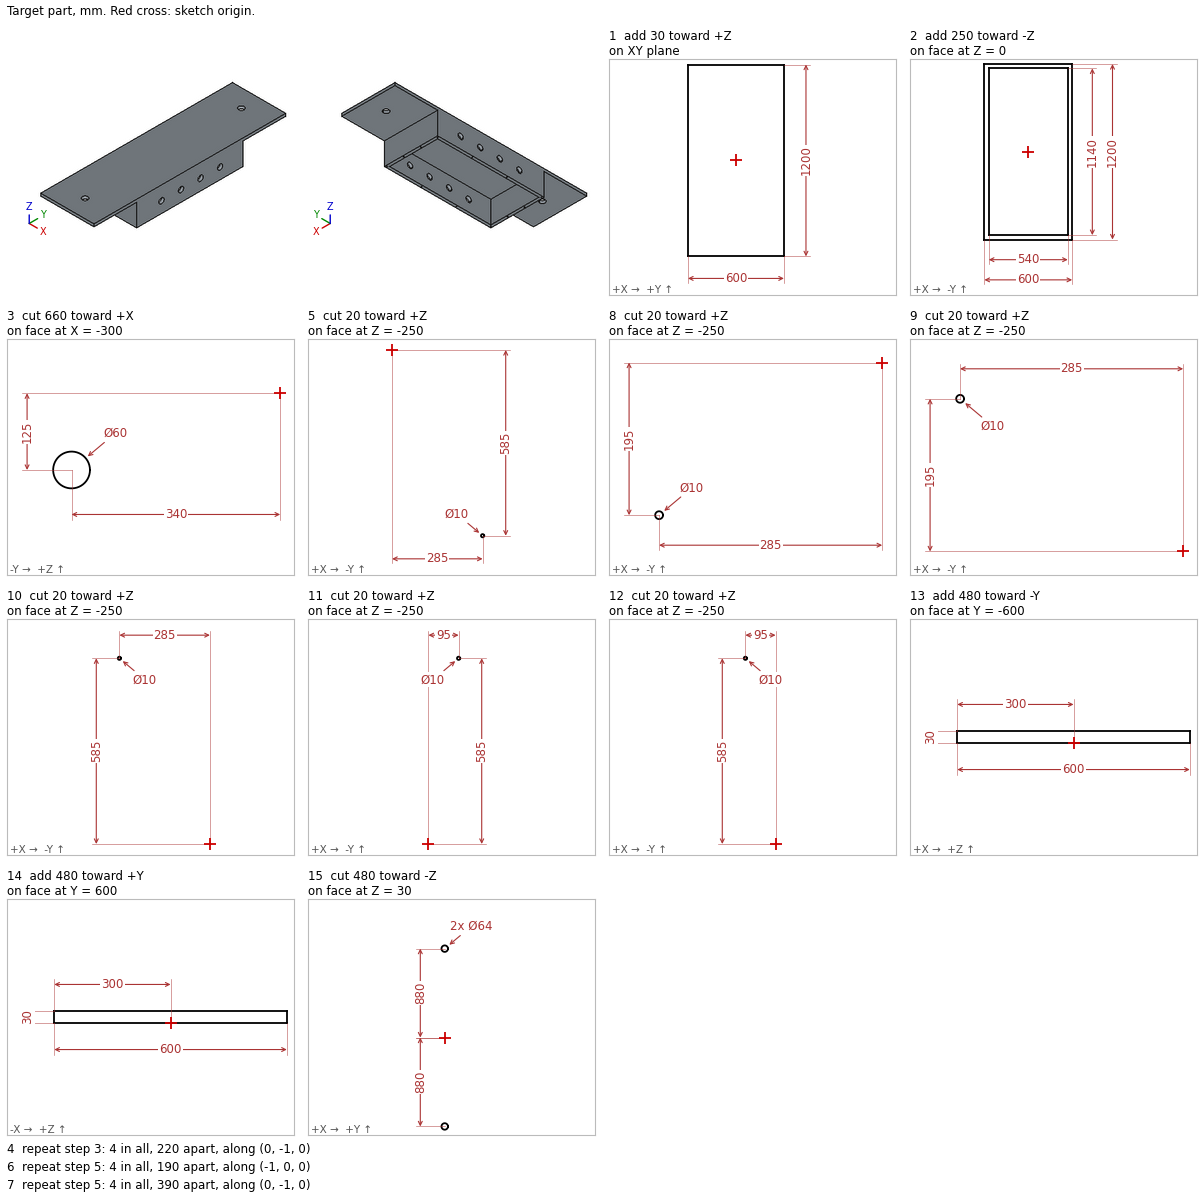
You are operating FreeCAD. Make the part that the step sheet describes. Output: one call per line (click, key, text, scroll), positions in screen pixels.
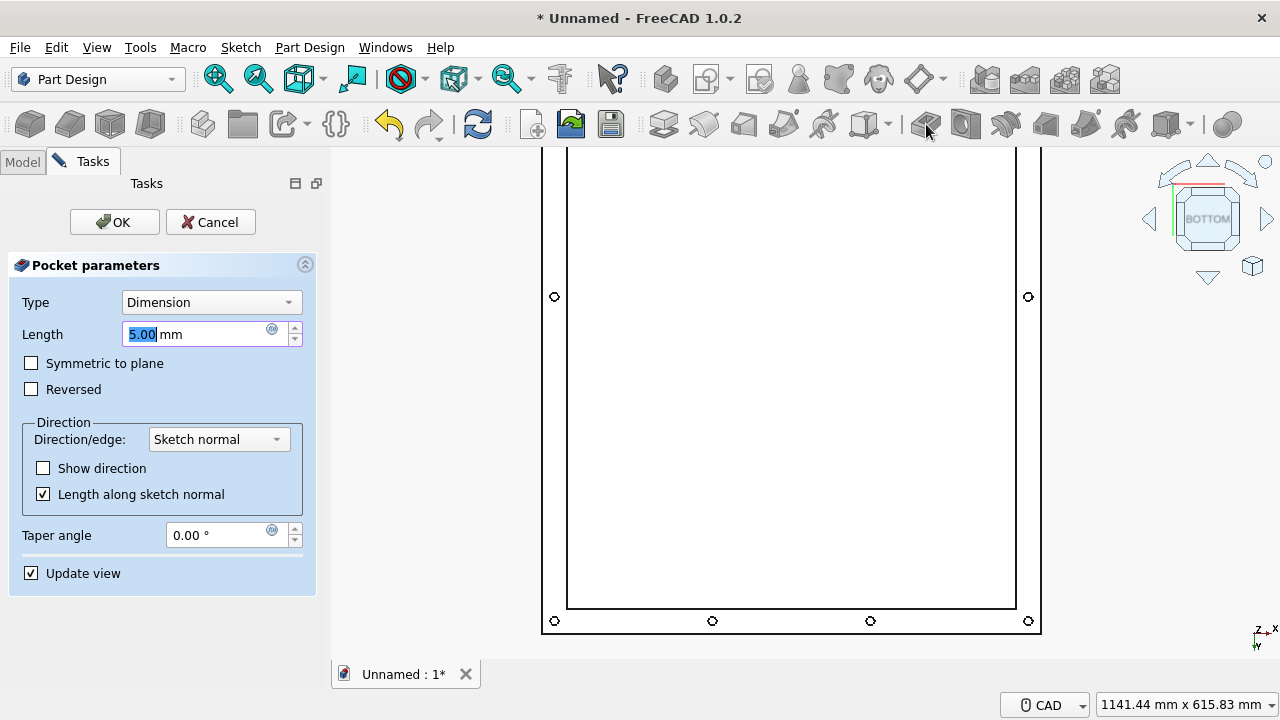
text(20)
key(Tab)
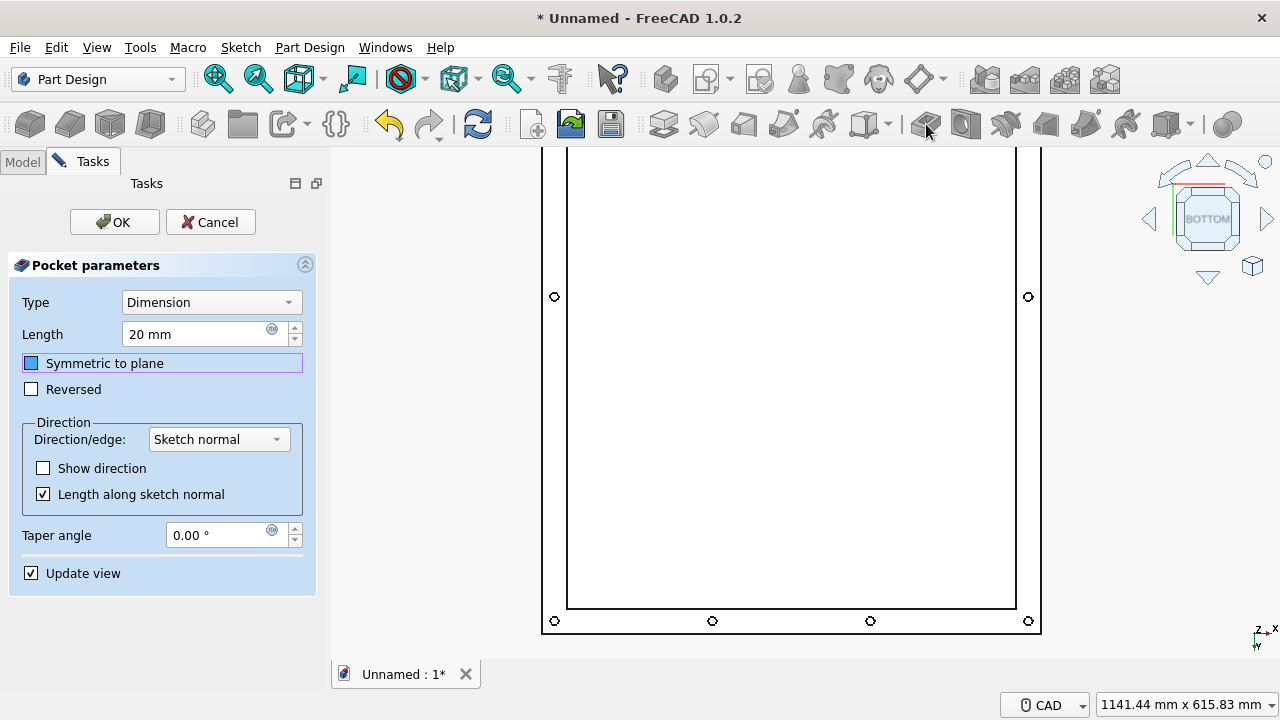
click(115, 222)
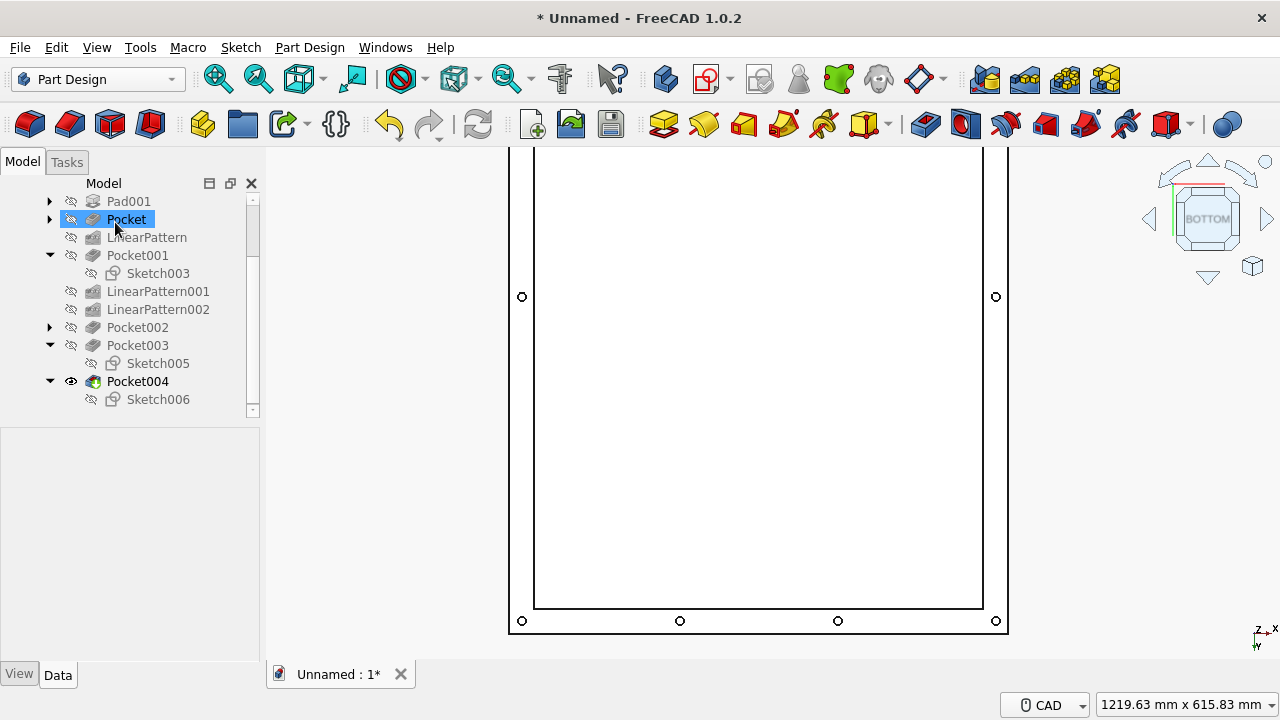
click(220, 80)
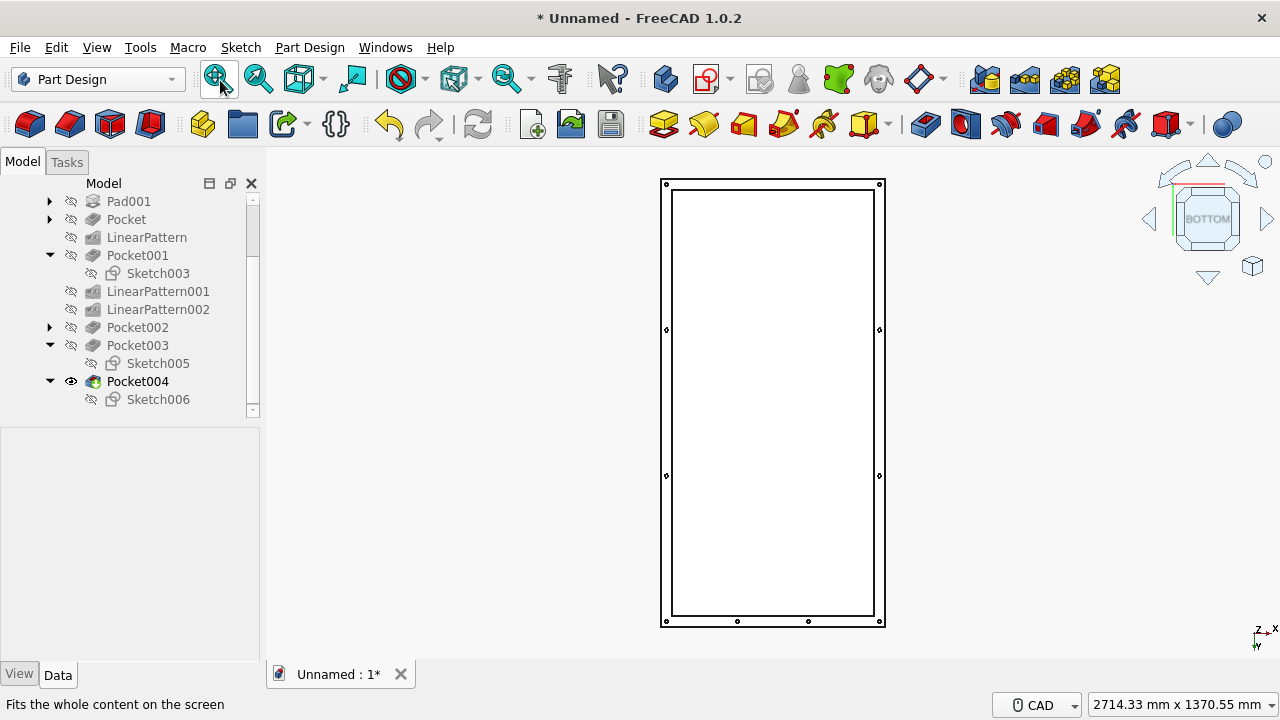
scroll(762, 620, up, 5)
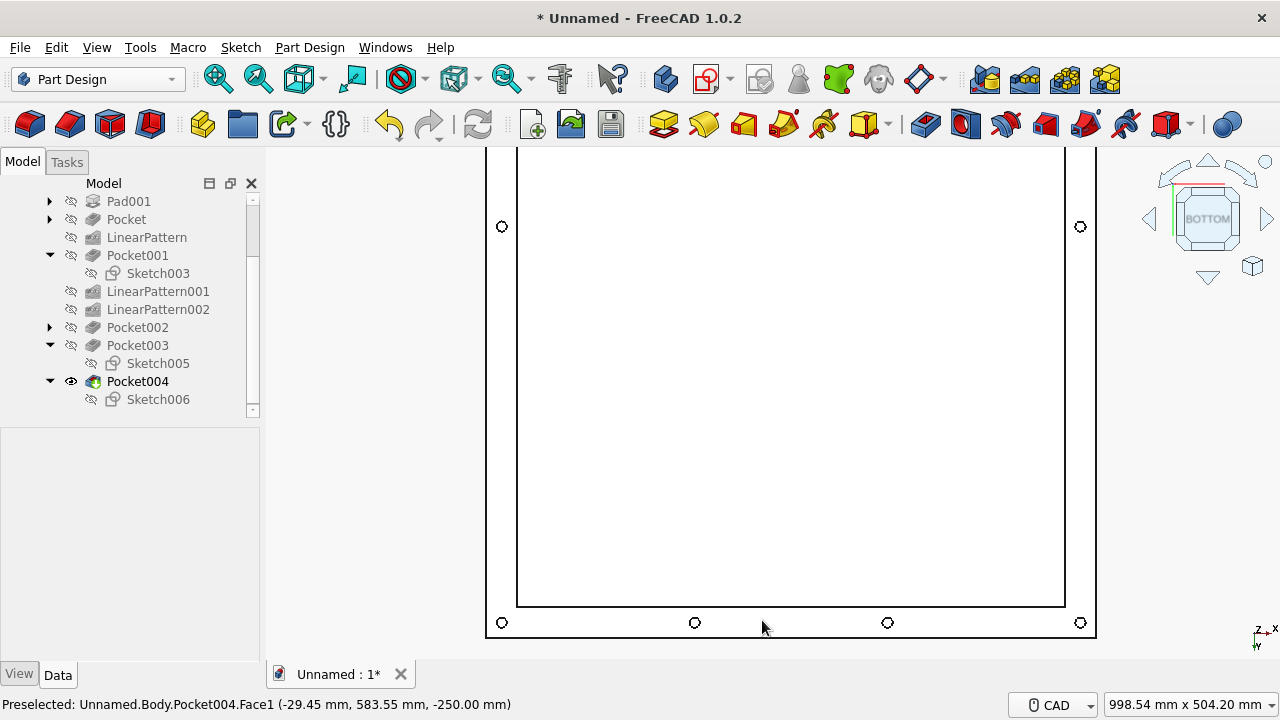
click(760, 621)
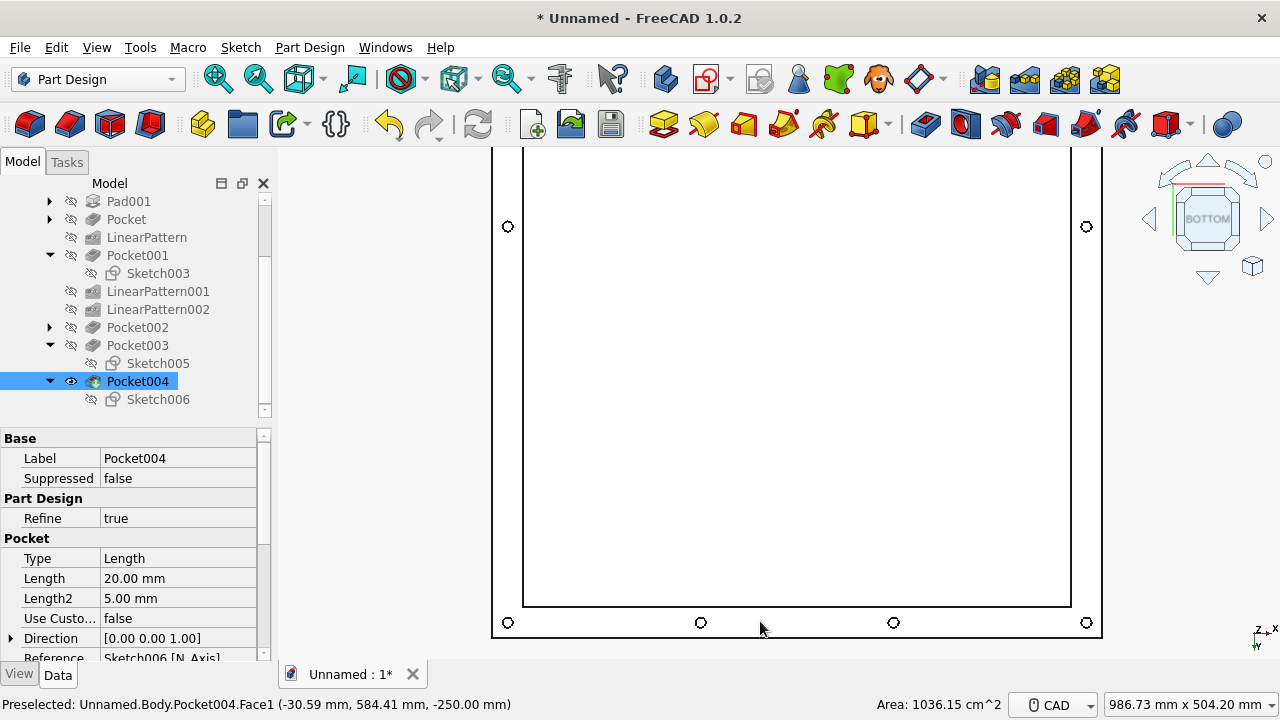
click(706, 80)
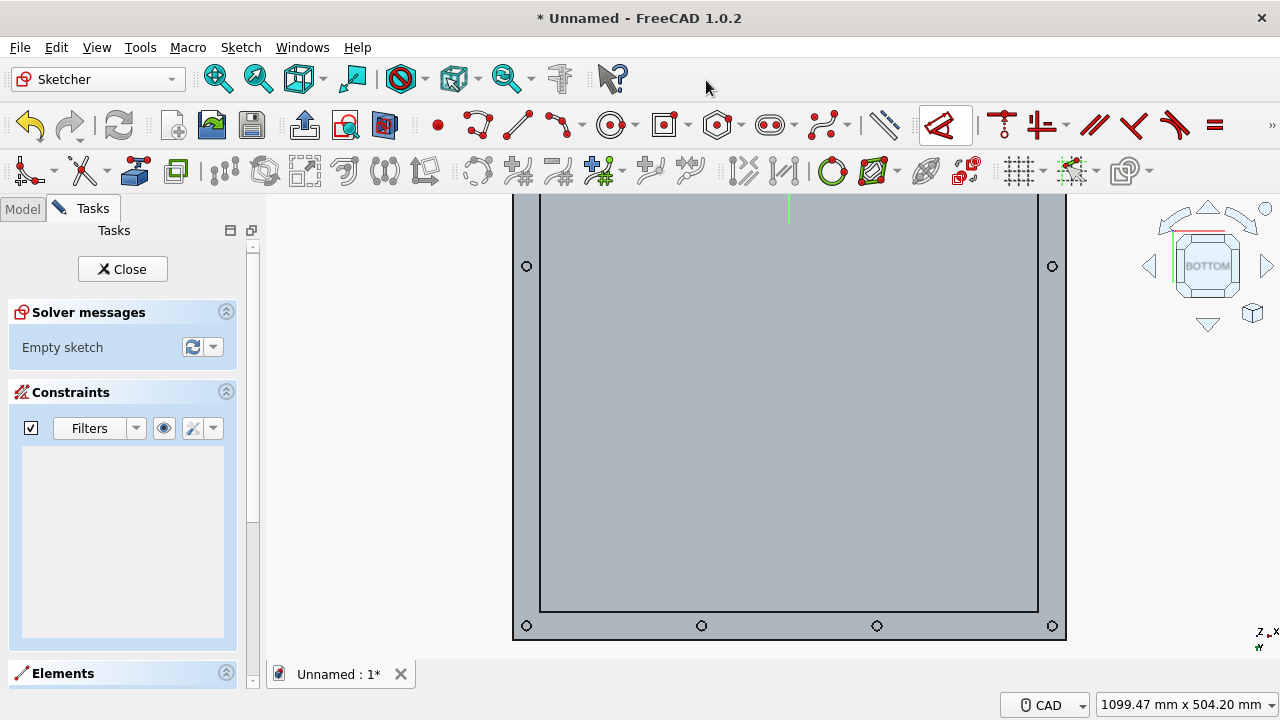
scroll(704, 426, down, 5)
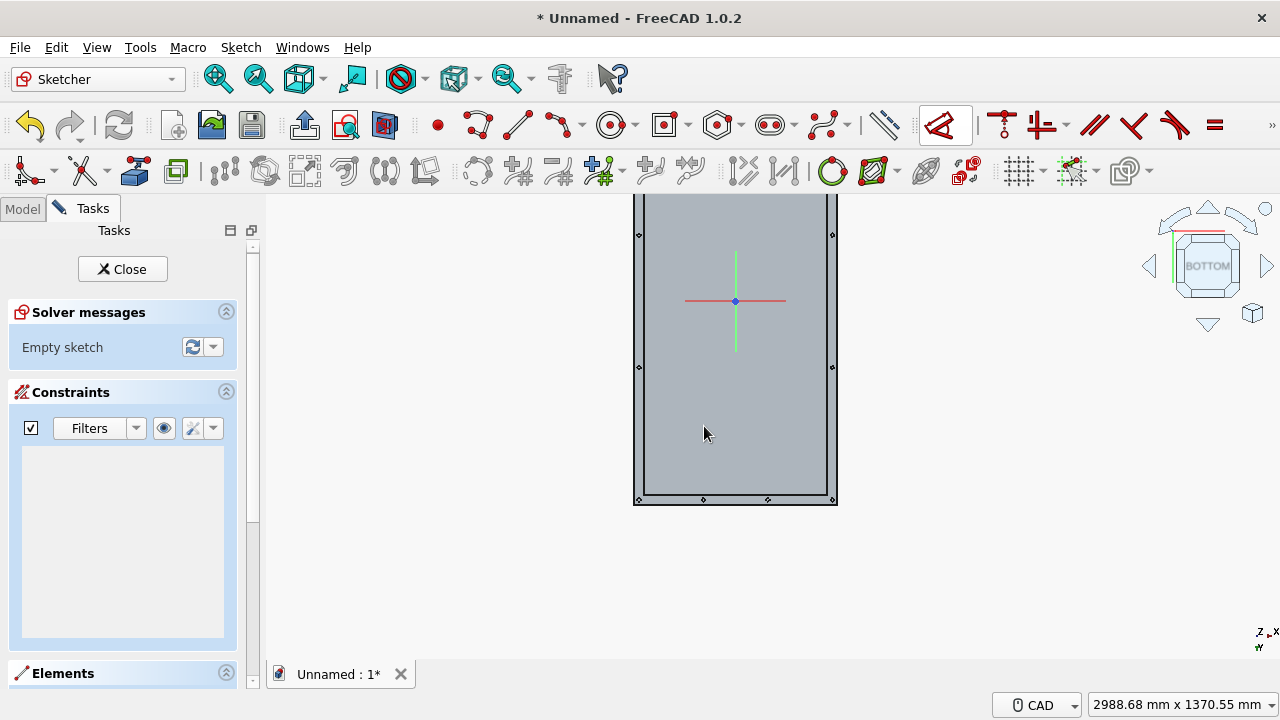
scroll(704, 426, down, 5)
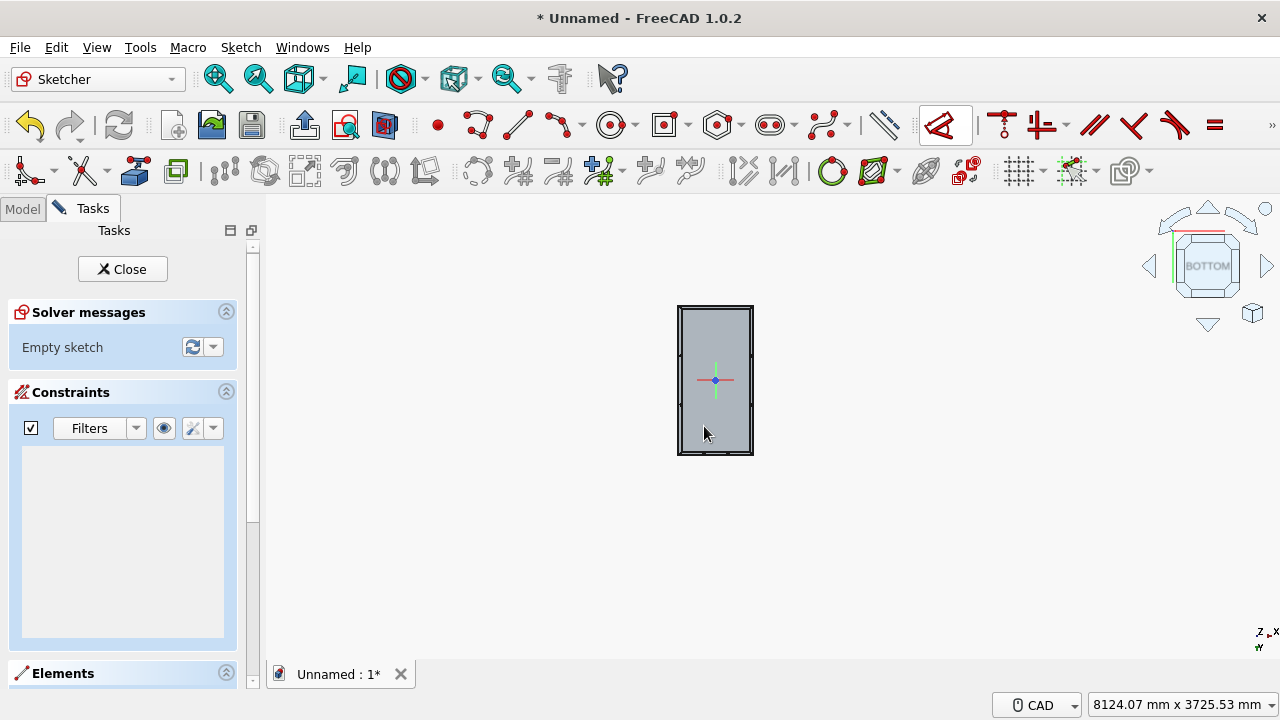
scroll(729, 301, up, 15)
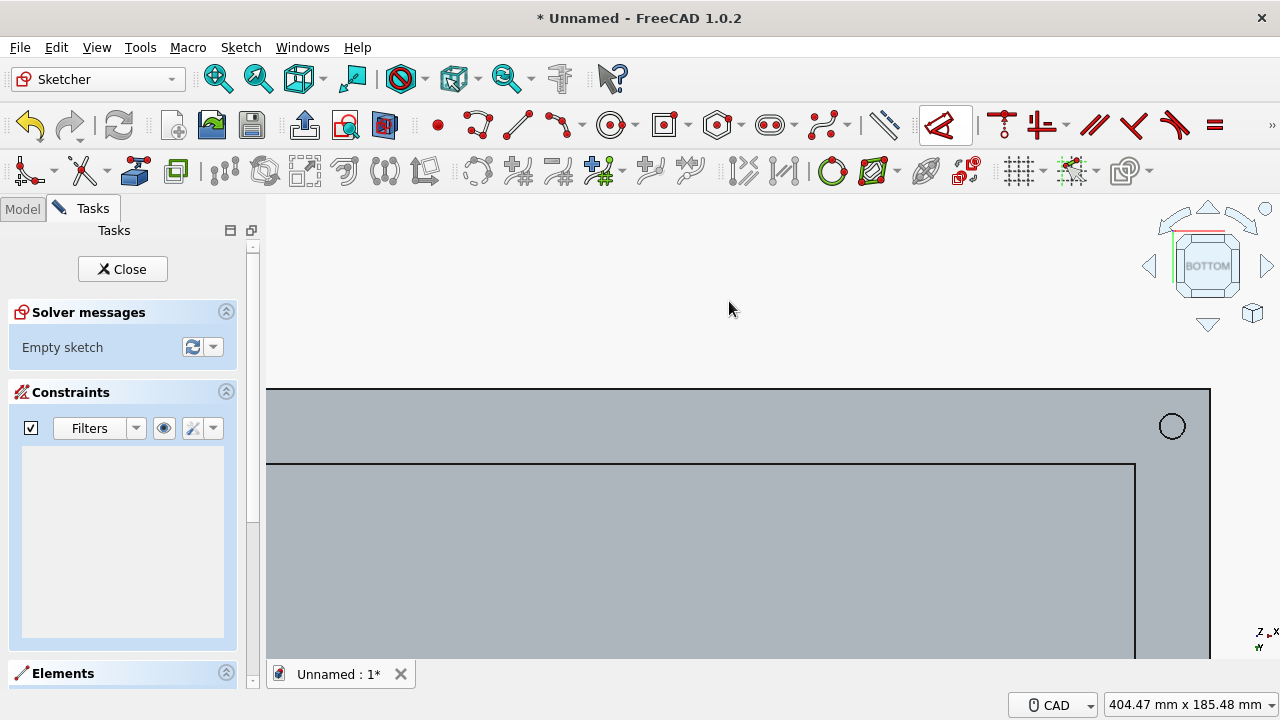
scroll(695, 426, up, 12)